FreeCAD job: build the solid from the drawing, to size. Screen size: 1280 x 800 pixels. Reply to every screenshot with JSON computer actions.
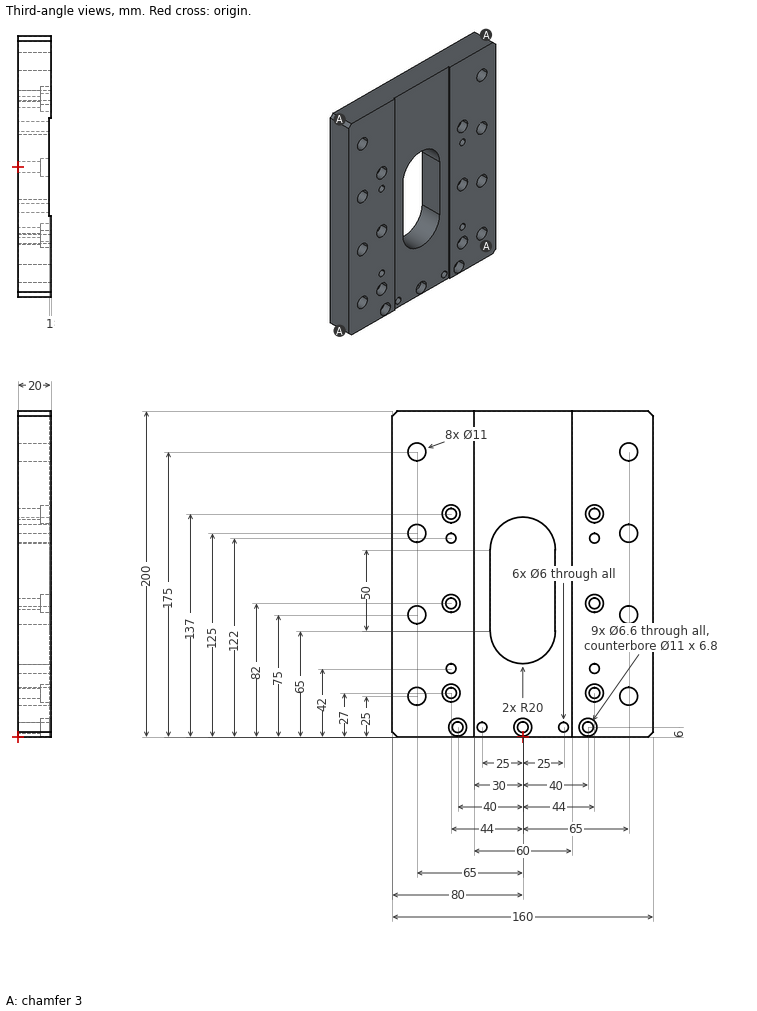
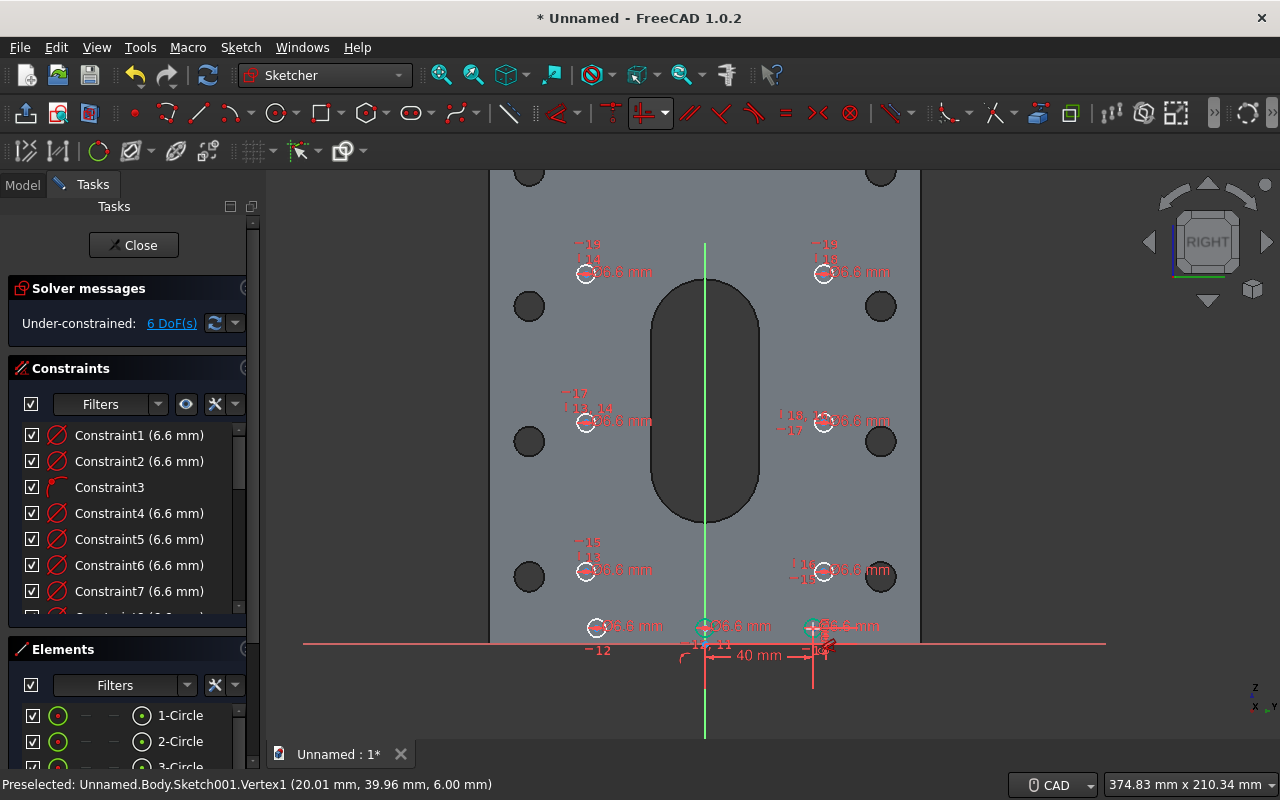
{"action": "left_click", "coordinate": [597, 628]}
{"action": "left_click", "coordinate": [651, 678]}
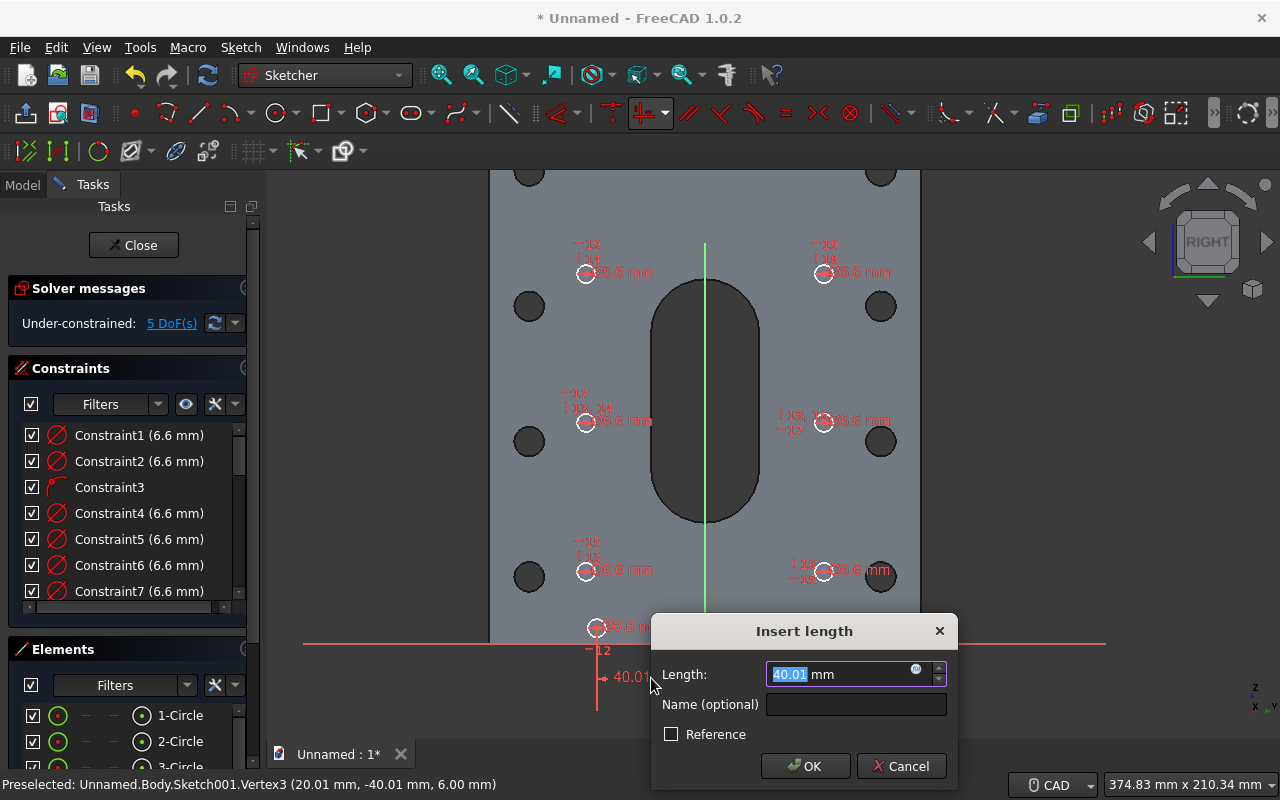
{"action": "type", "text": "40"}
{"action": "key", "text": "Return"}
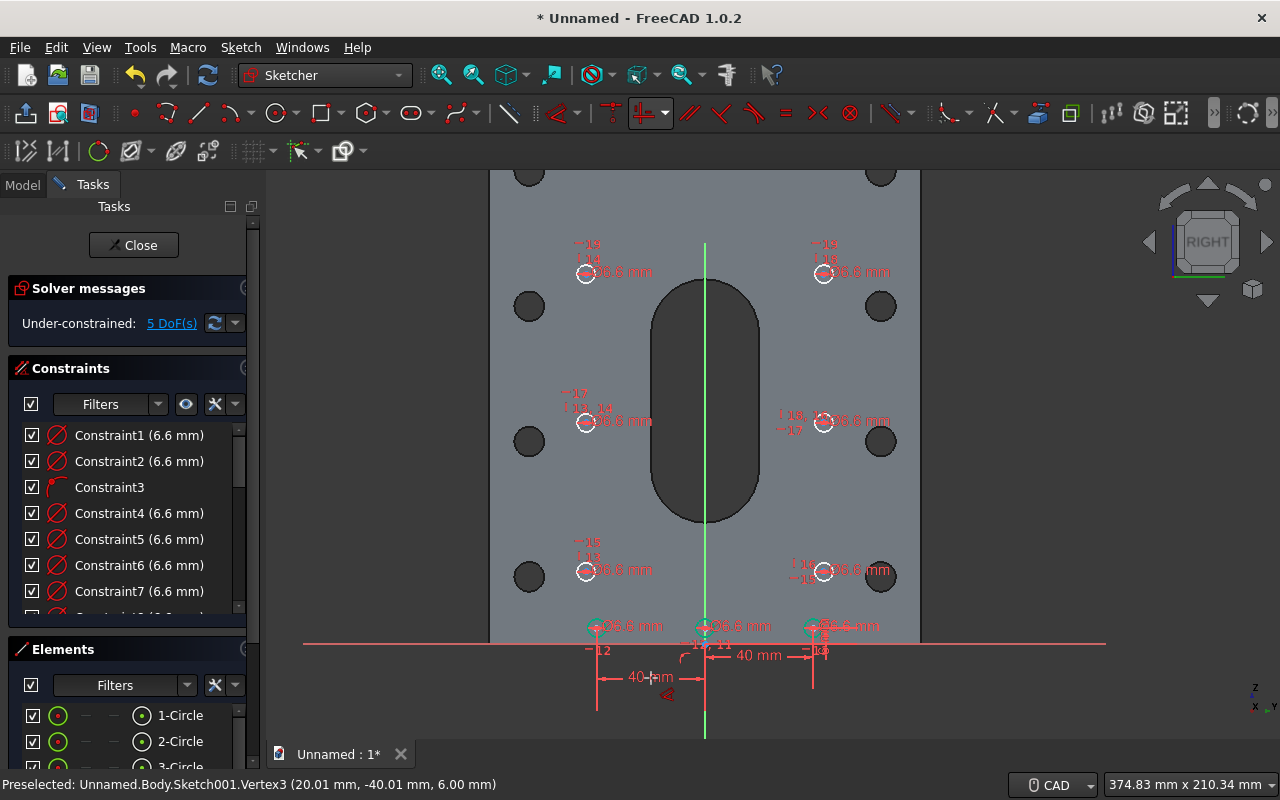
{"action": "left_click", "coordinate": [586, 572]}
{"action": "left_click", "coordinate": [646, 538]}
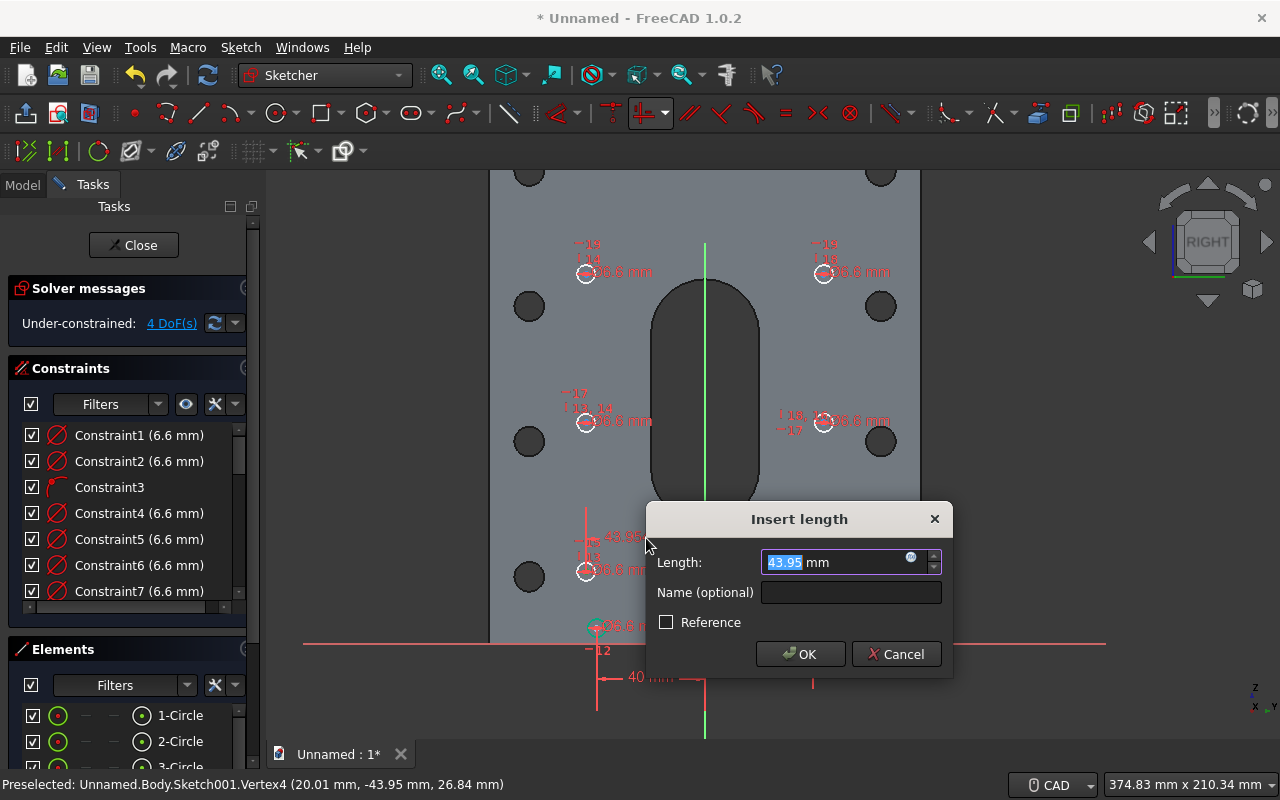
{"action": "type", "text": "44"}
{"action": "key", "text": "Return"}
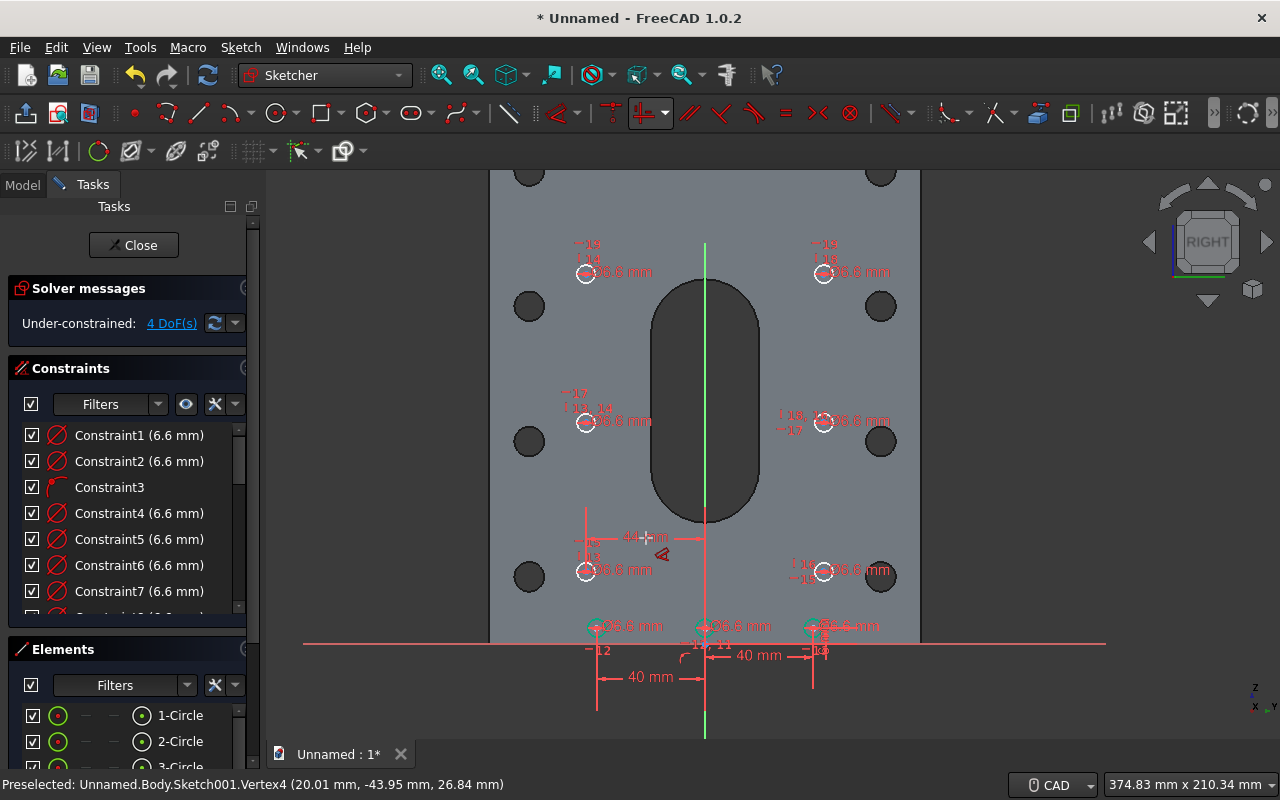
{"action": "left_click", "coordinate": [586, 572]}
{"action": "left_click", "coordinate": [552, 608]}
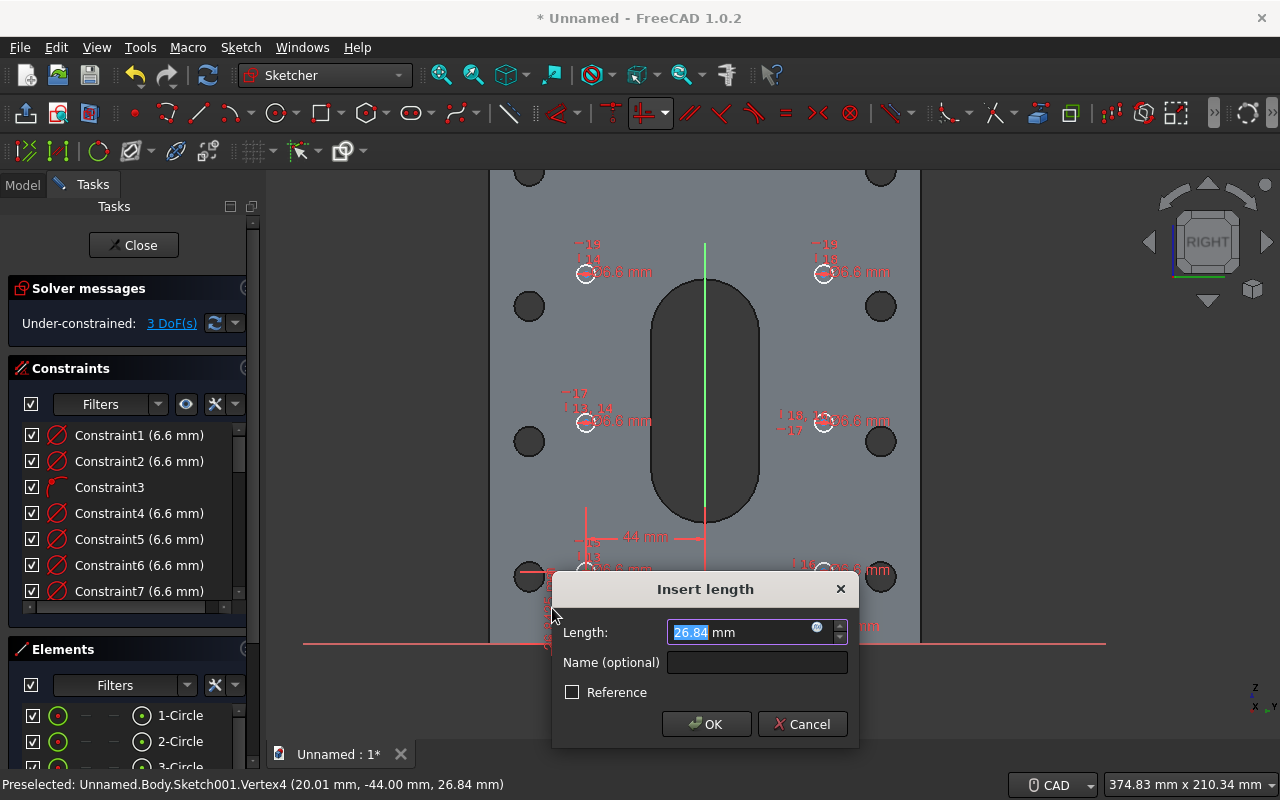
{"action": "type", "text": "27"}
{"action": "key", "text": "Return"}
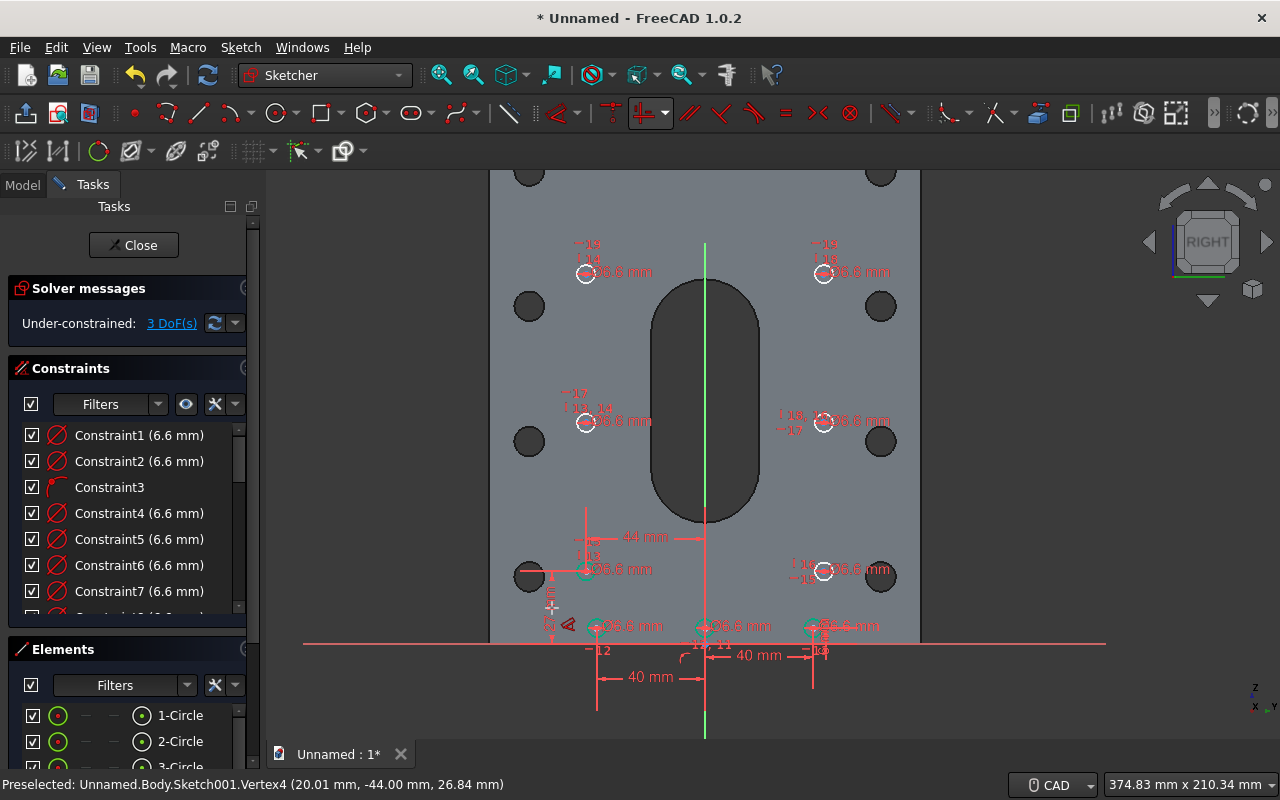
{"action": "left_click", "coordinate": [586, 423]}
{"action": "left_click", "coordinate": [552, 534]}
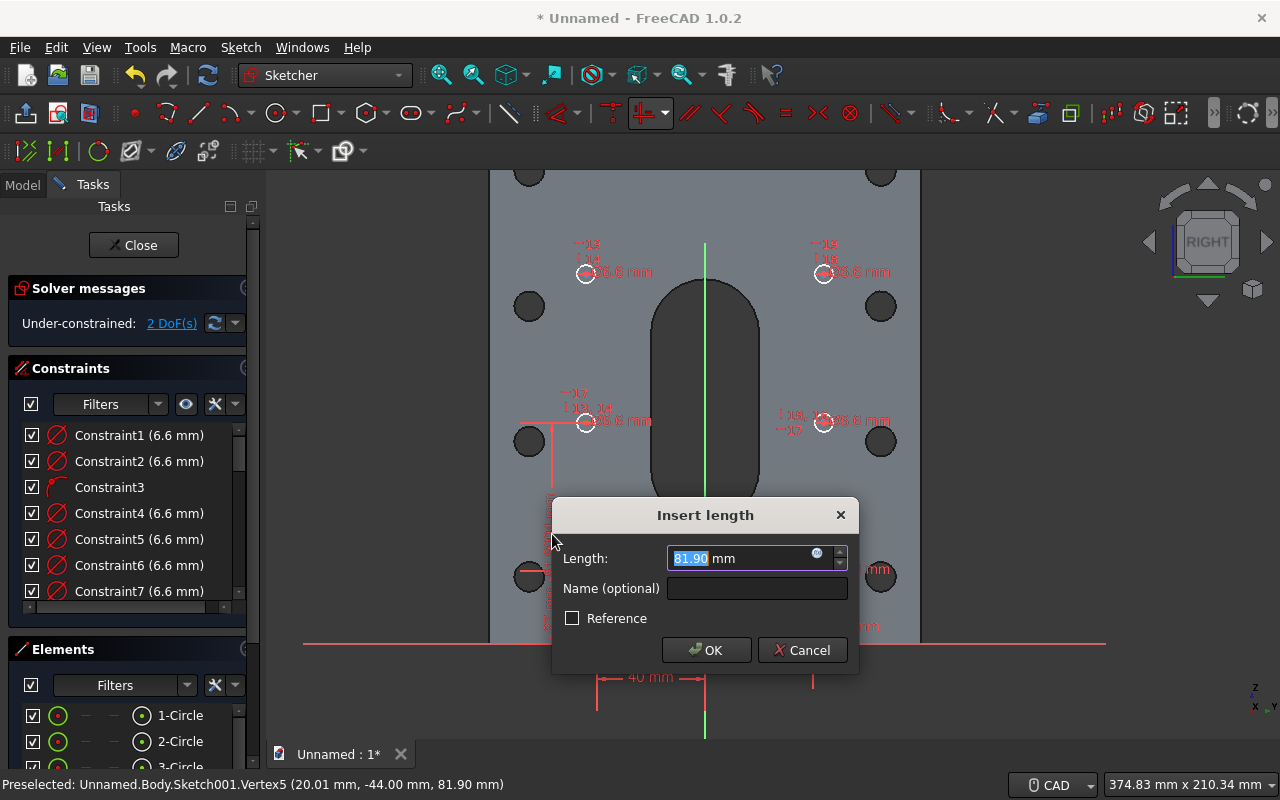
{"action": "type", "text": "82"}
{"action": "key", "text": "Return"}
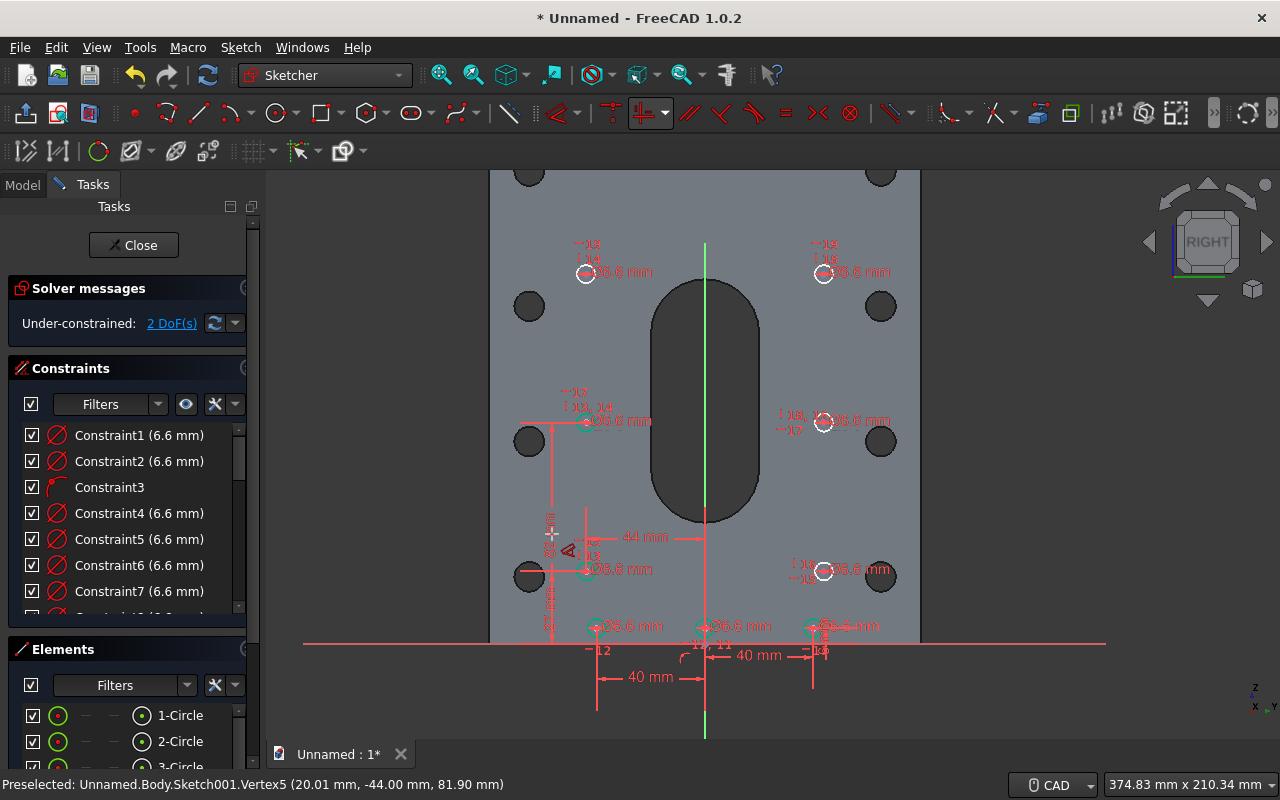
{"action": "left_click", "coordinate": [824, 571]}
{"action": "left_click", "coordinate": [765, 678]}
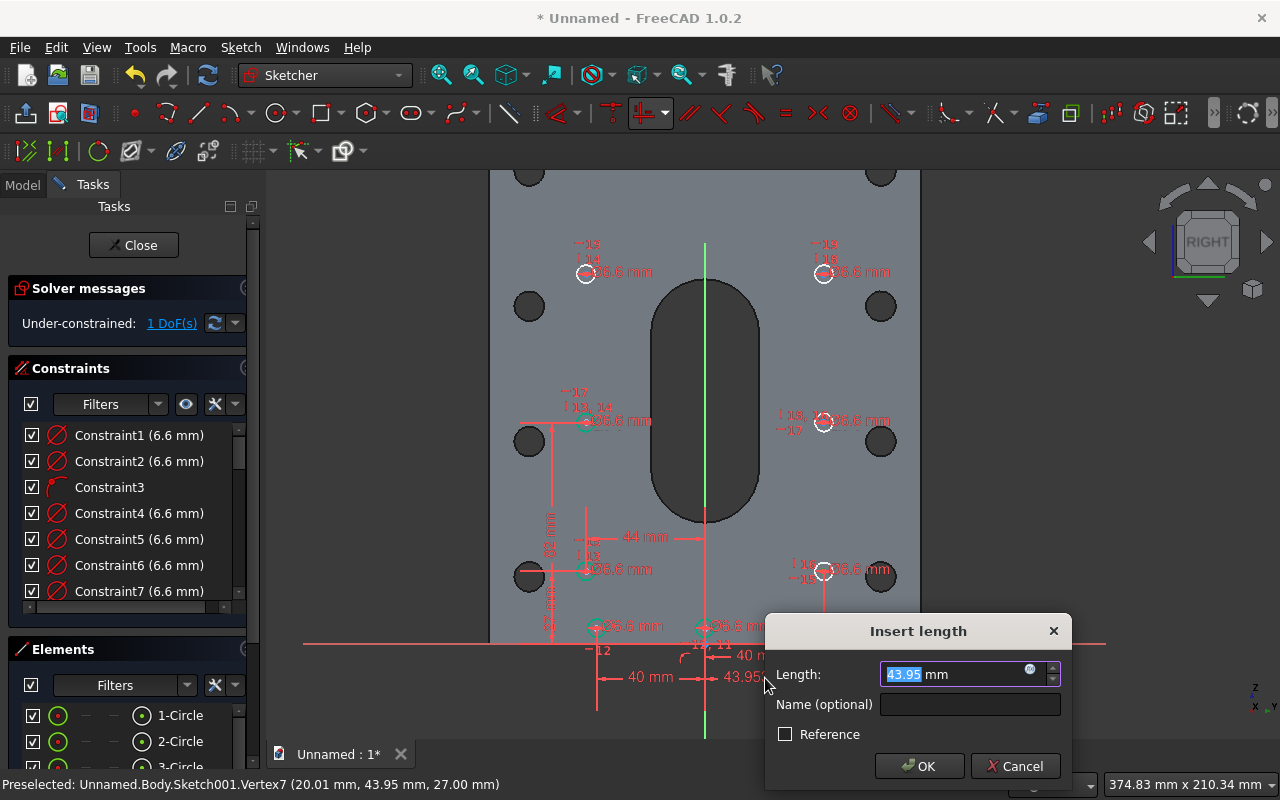
{"action": "type", "text": "44"}
{"action": "key", "text": "Return"}